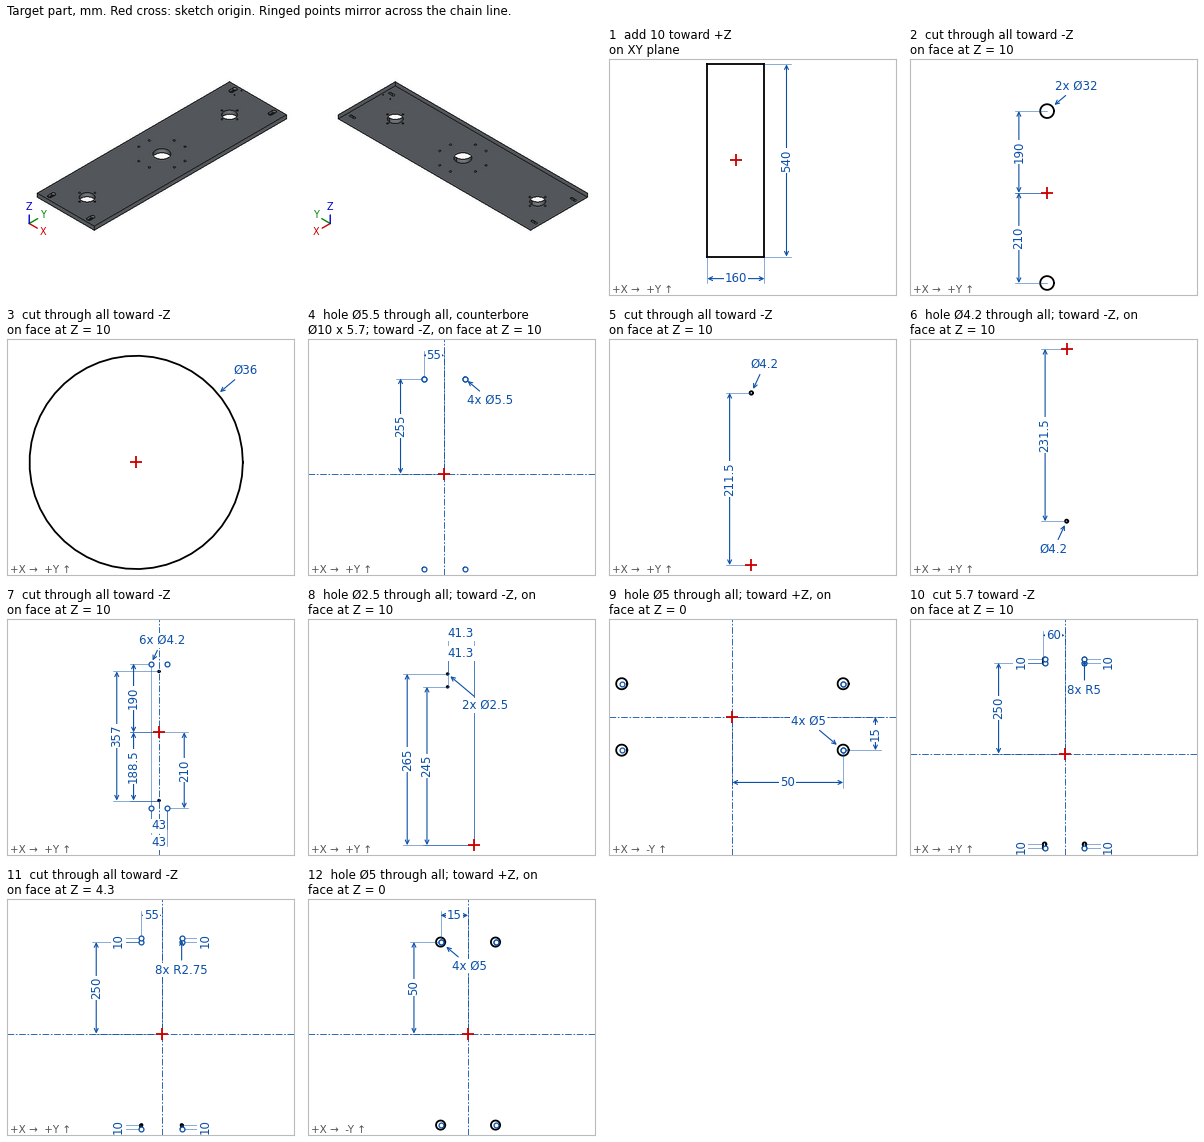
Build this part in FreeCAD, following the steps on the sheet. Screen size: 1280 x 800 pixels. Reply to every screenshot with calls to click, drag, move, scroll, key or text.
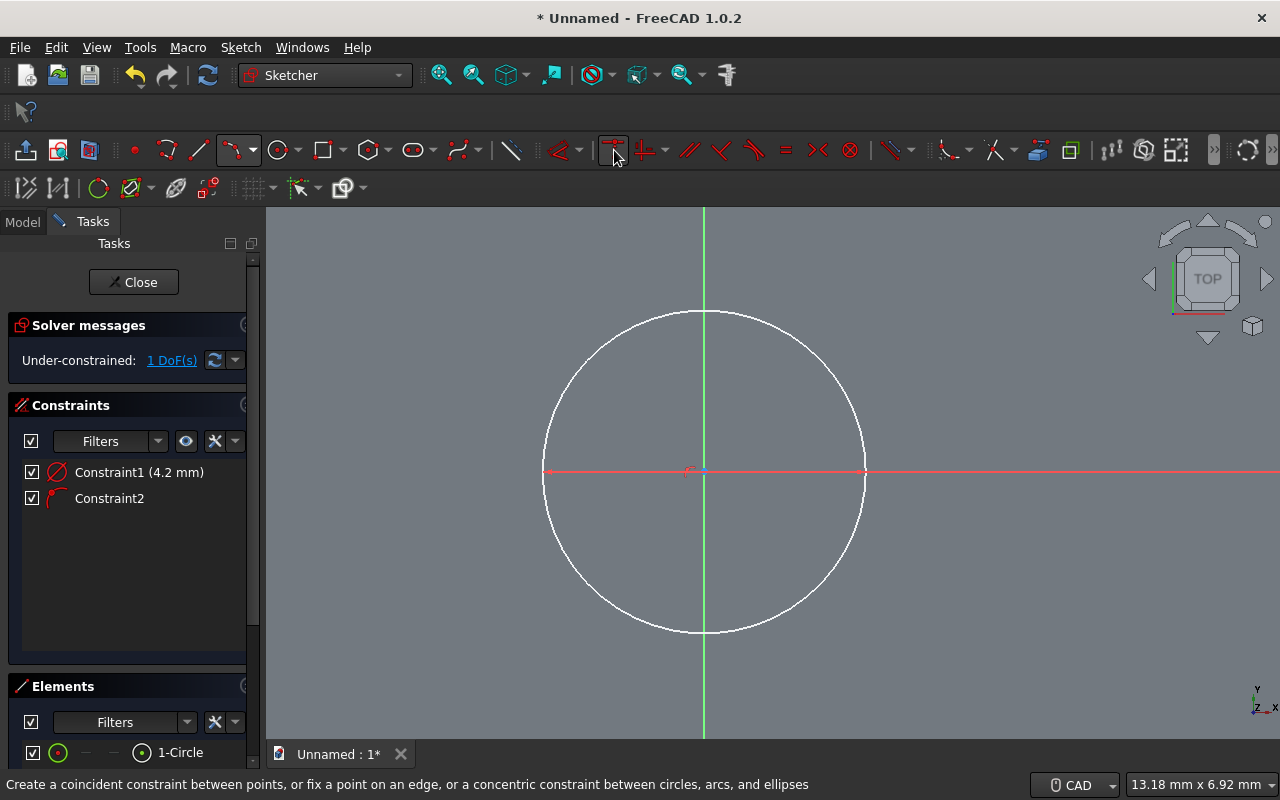
key(d)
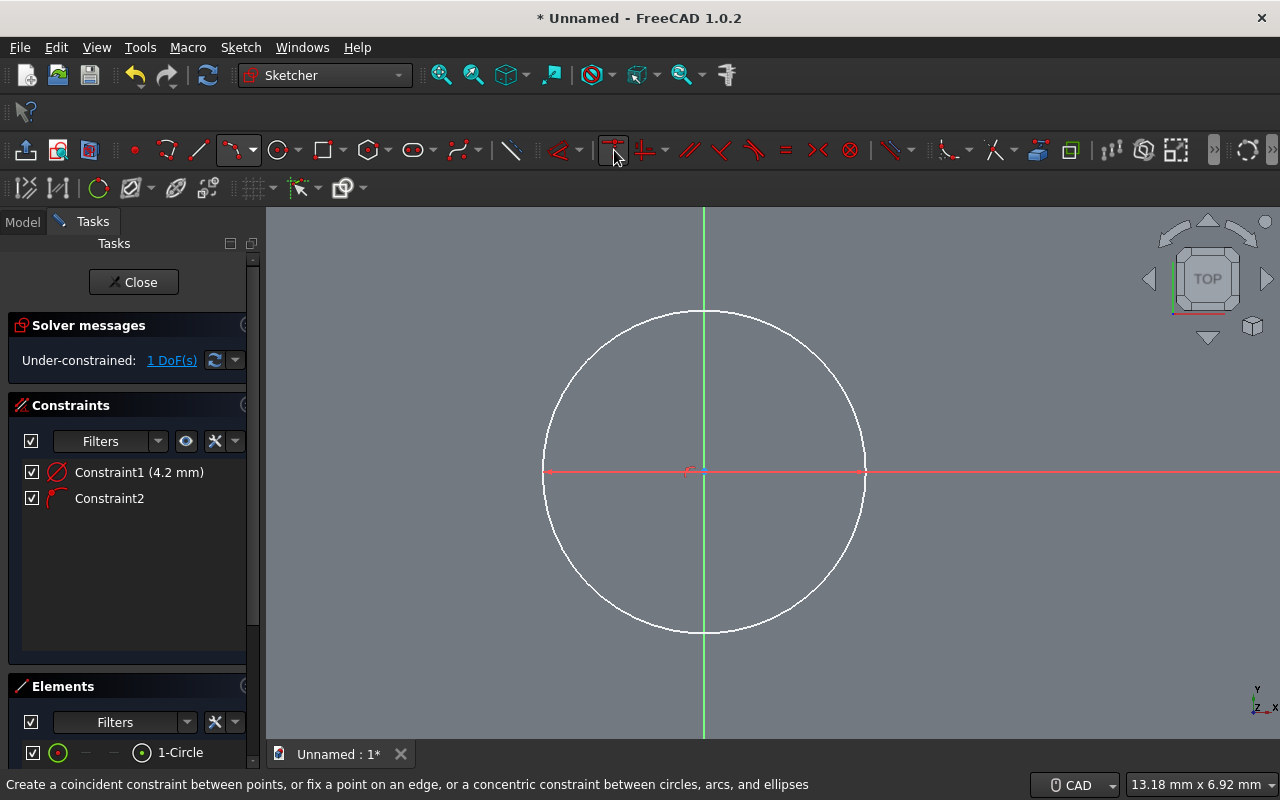
click(704, 472)
click(738, 591)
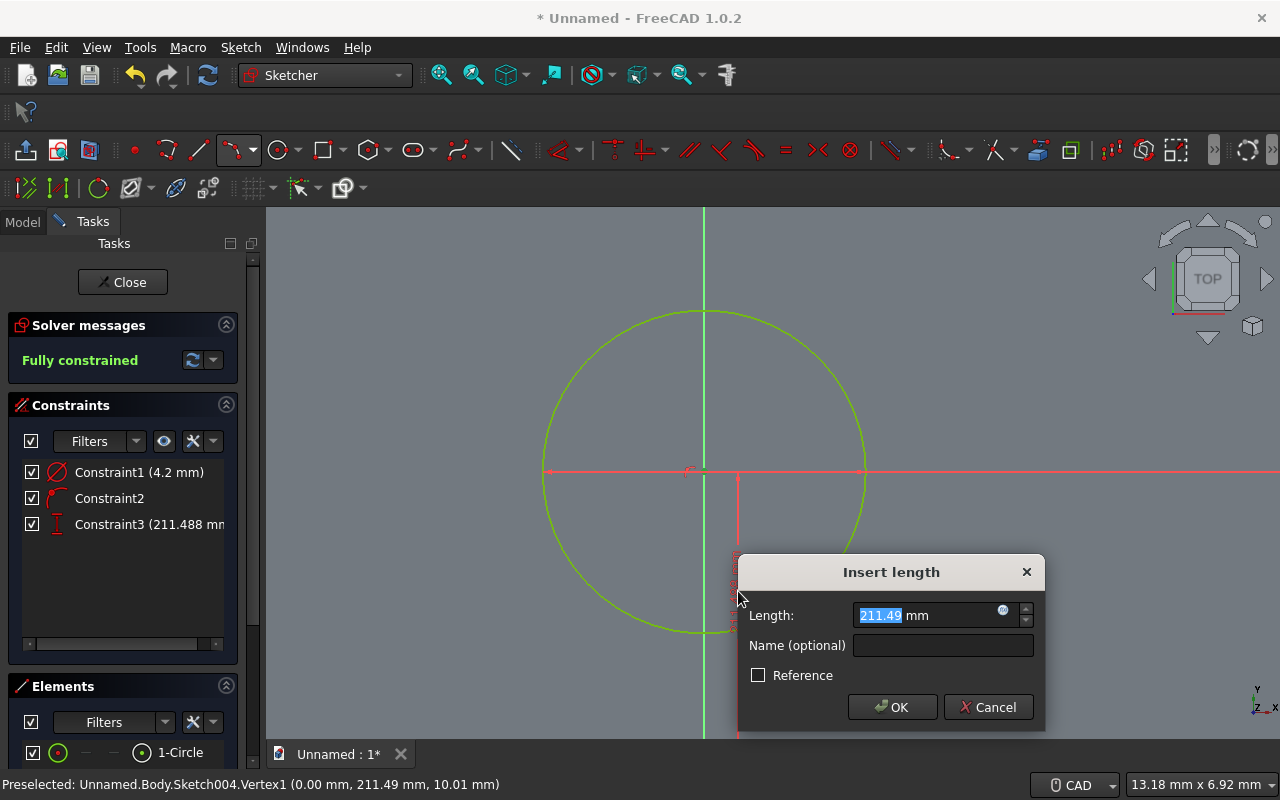
text(211.5)
key(Return)
key(Escape)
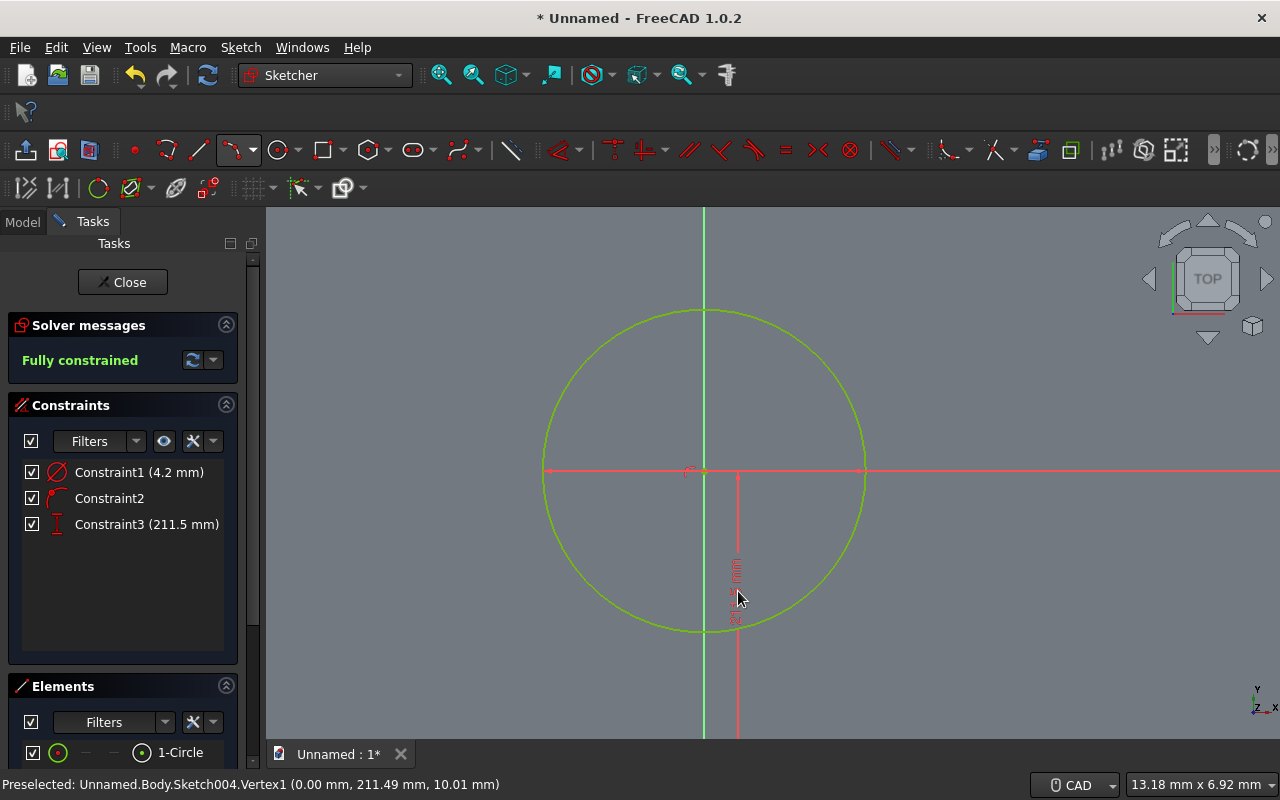
click(123, 282)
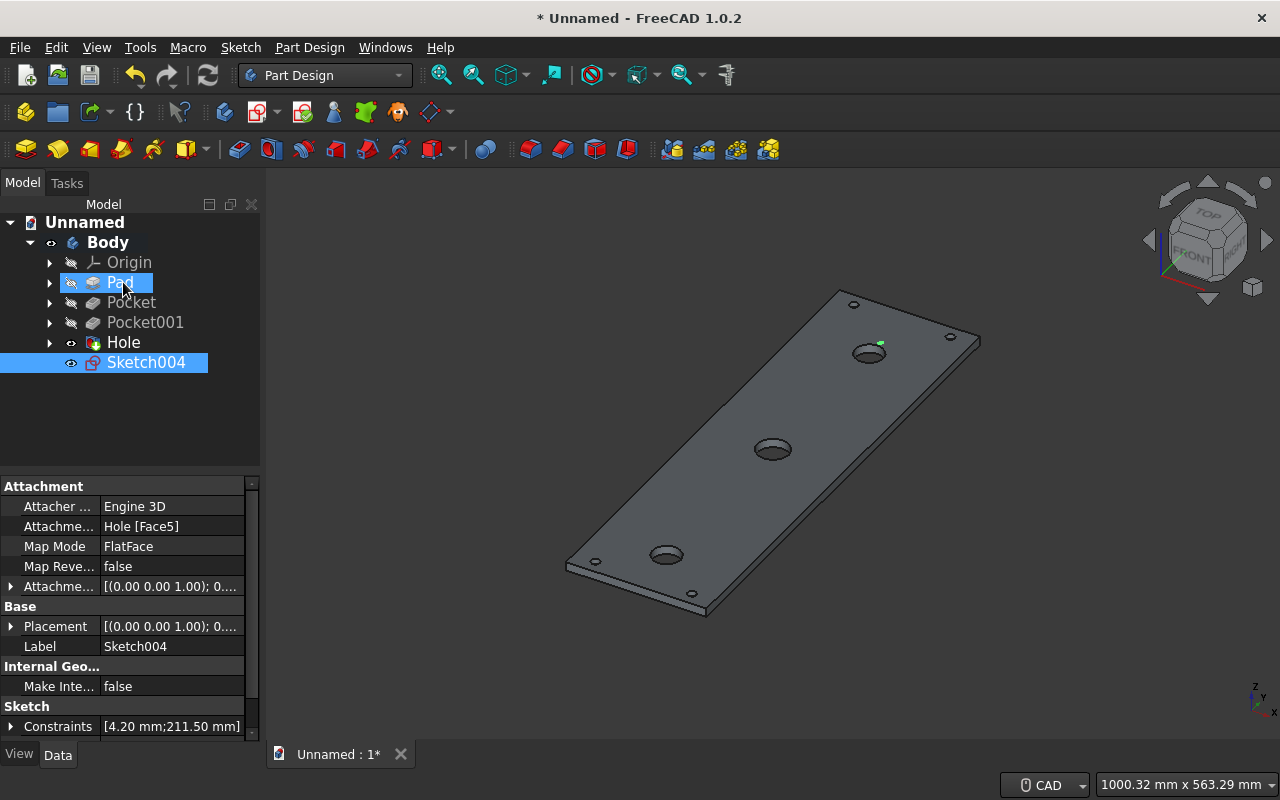
click(240, 150)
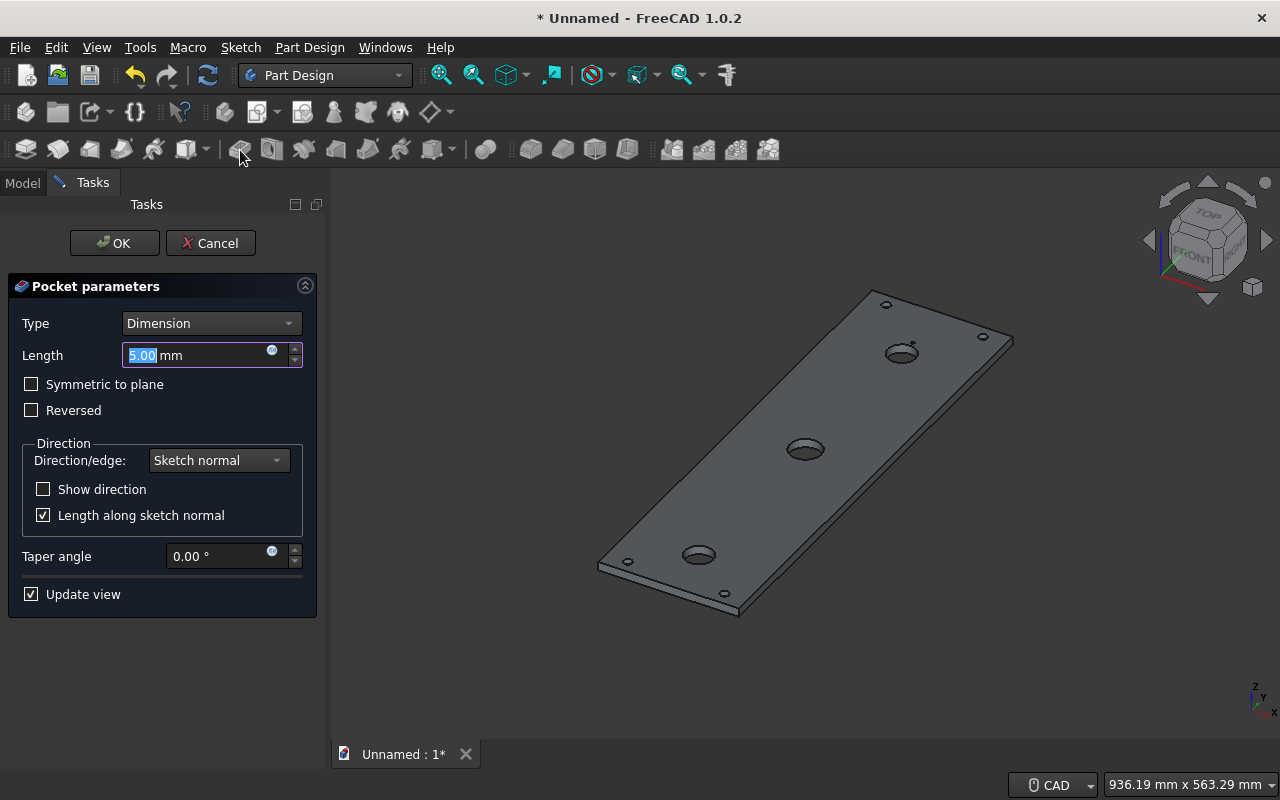
click(212, 324)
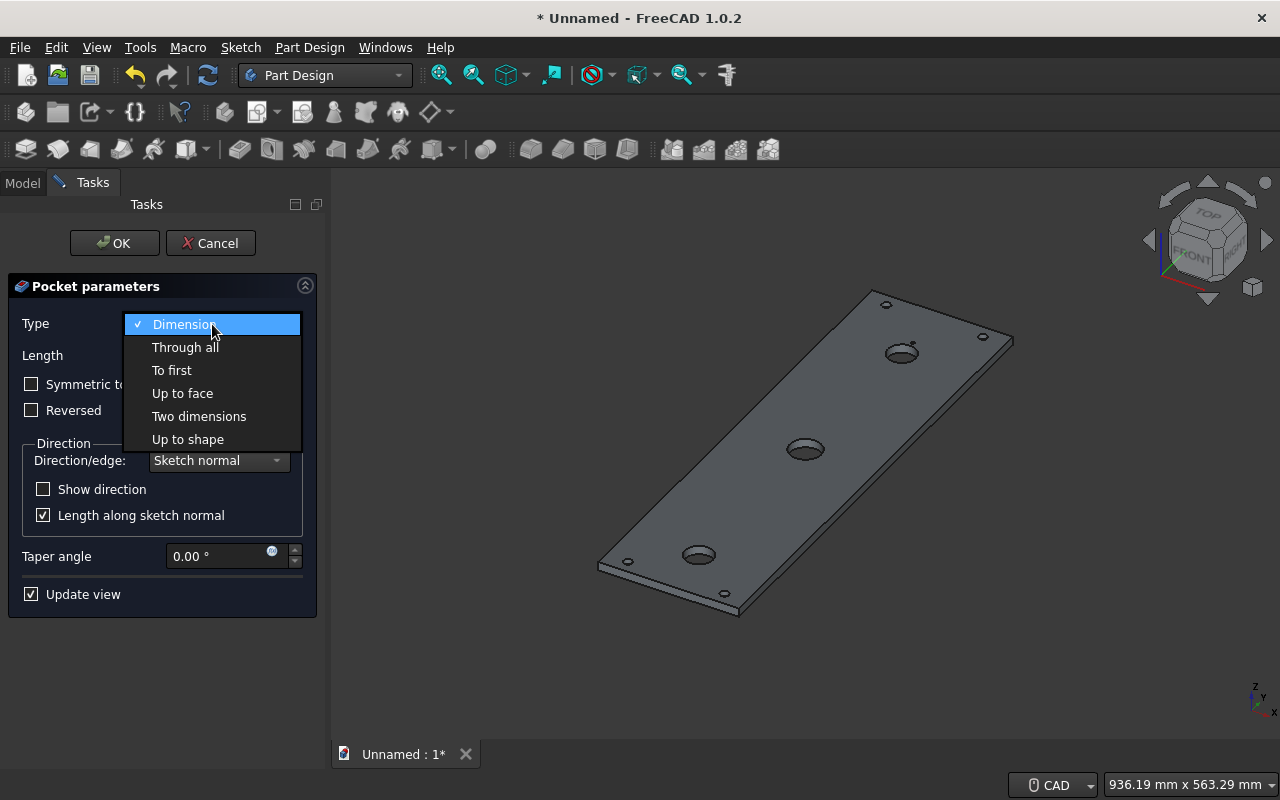
click(212, 348)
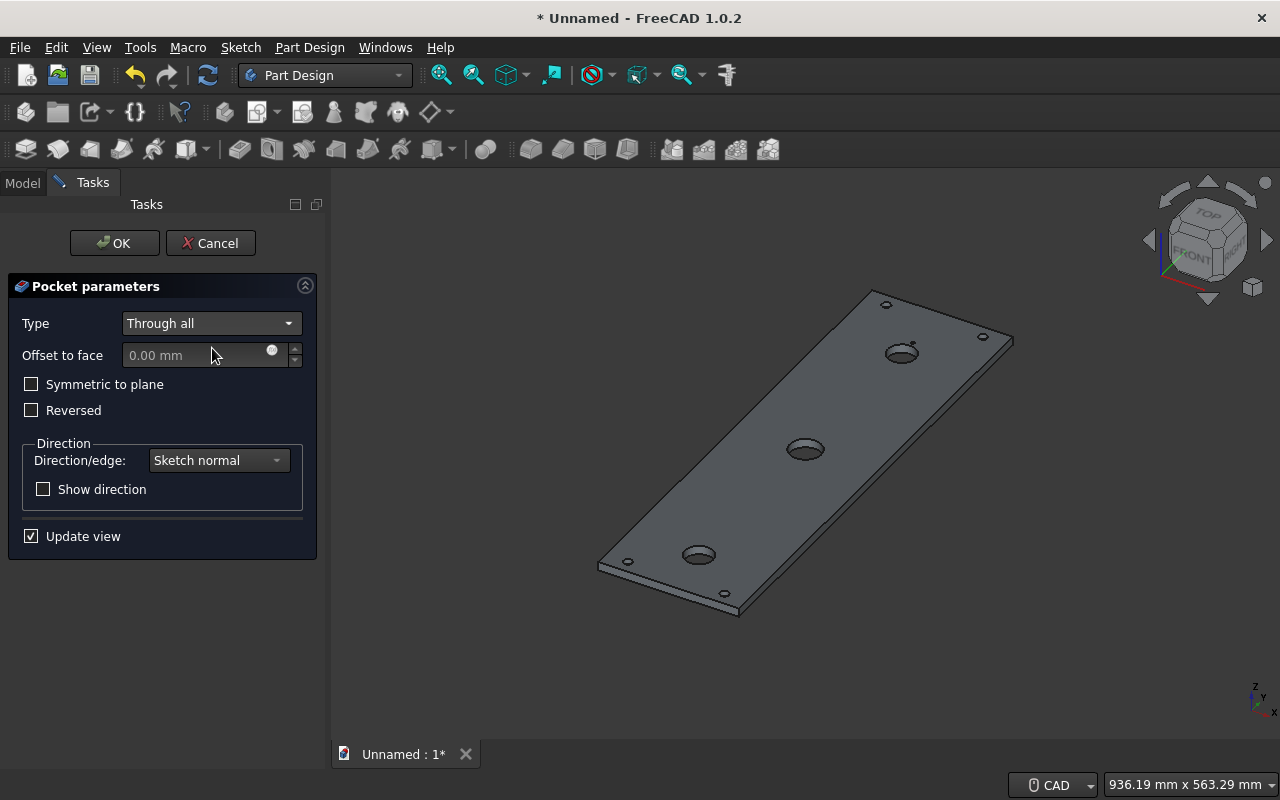
click(115, 243)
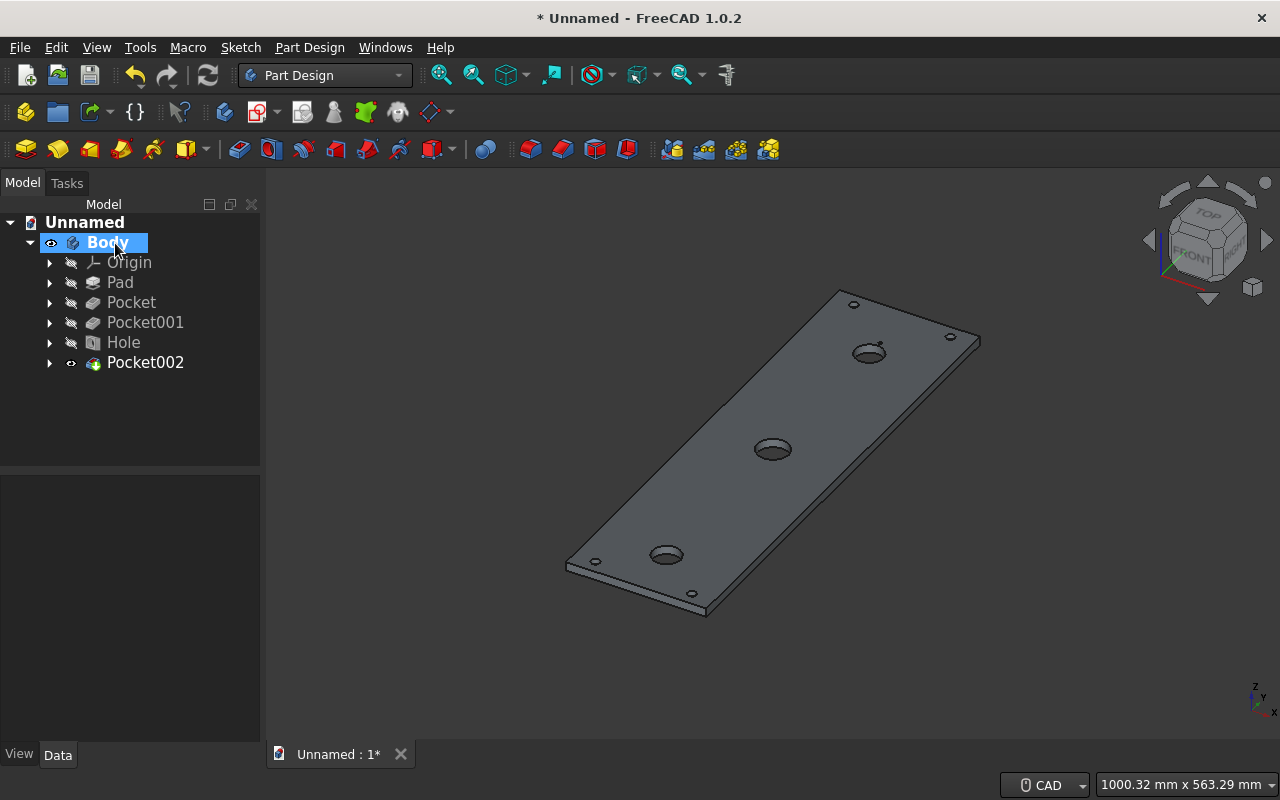
click(812, 410)